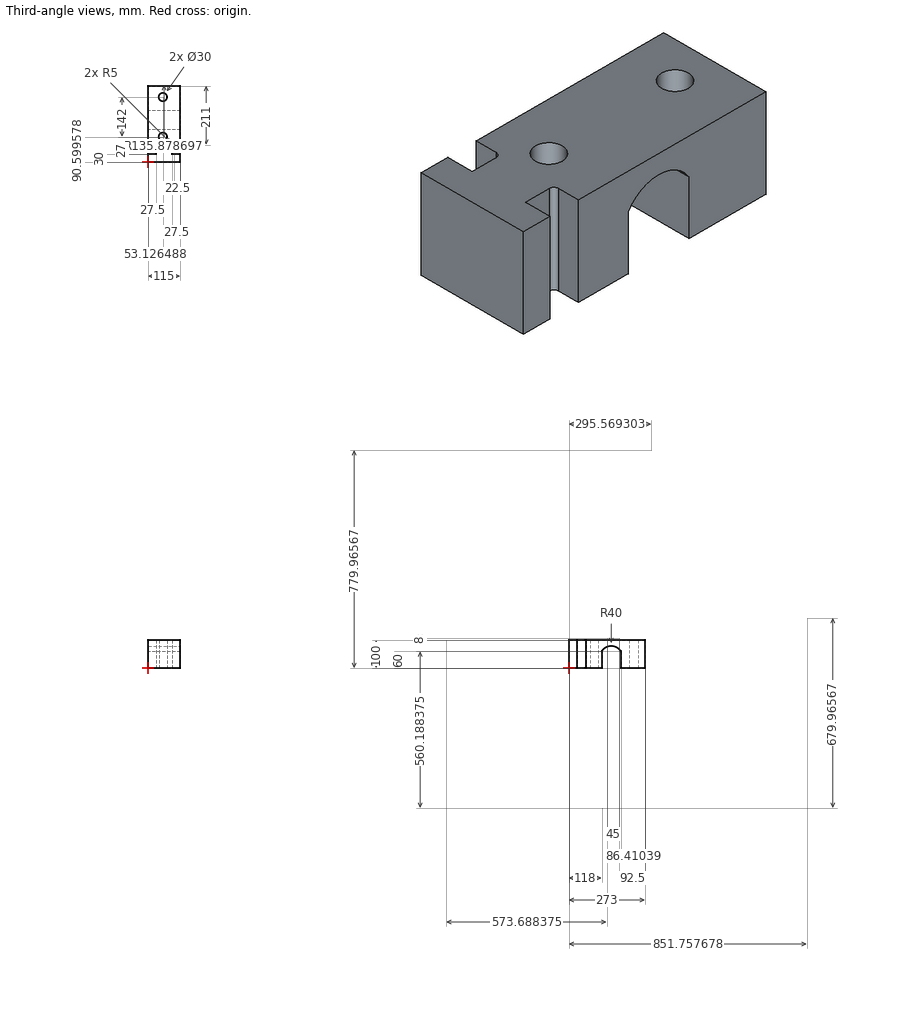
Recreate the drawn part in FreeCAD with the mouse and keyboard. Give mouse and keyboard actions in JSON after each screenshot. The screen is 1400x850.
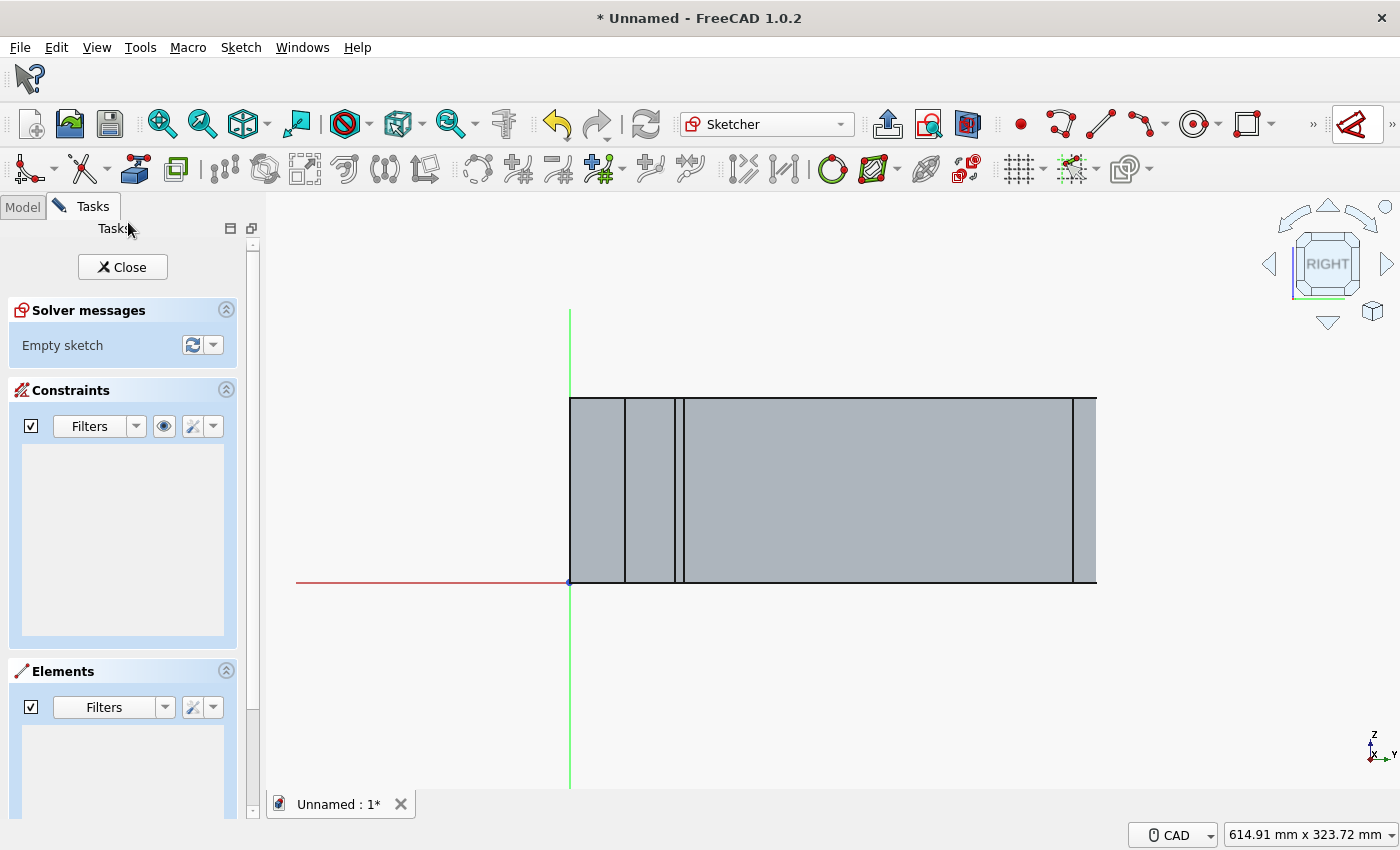
{"action": "key", "text": "q s"}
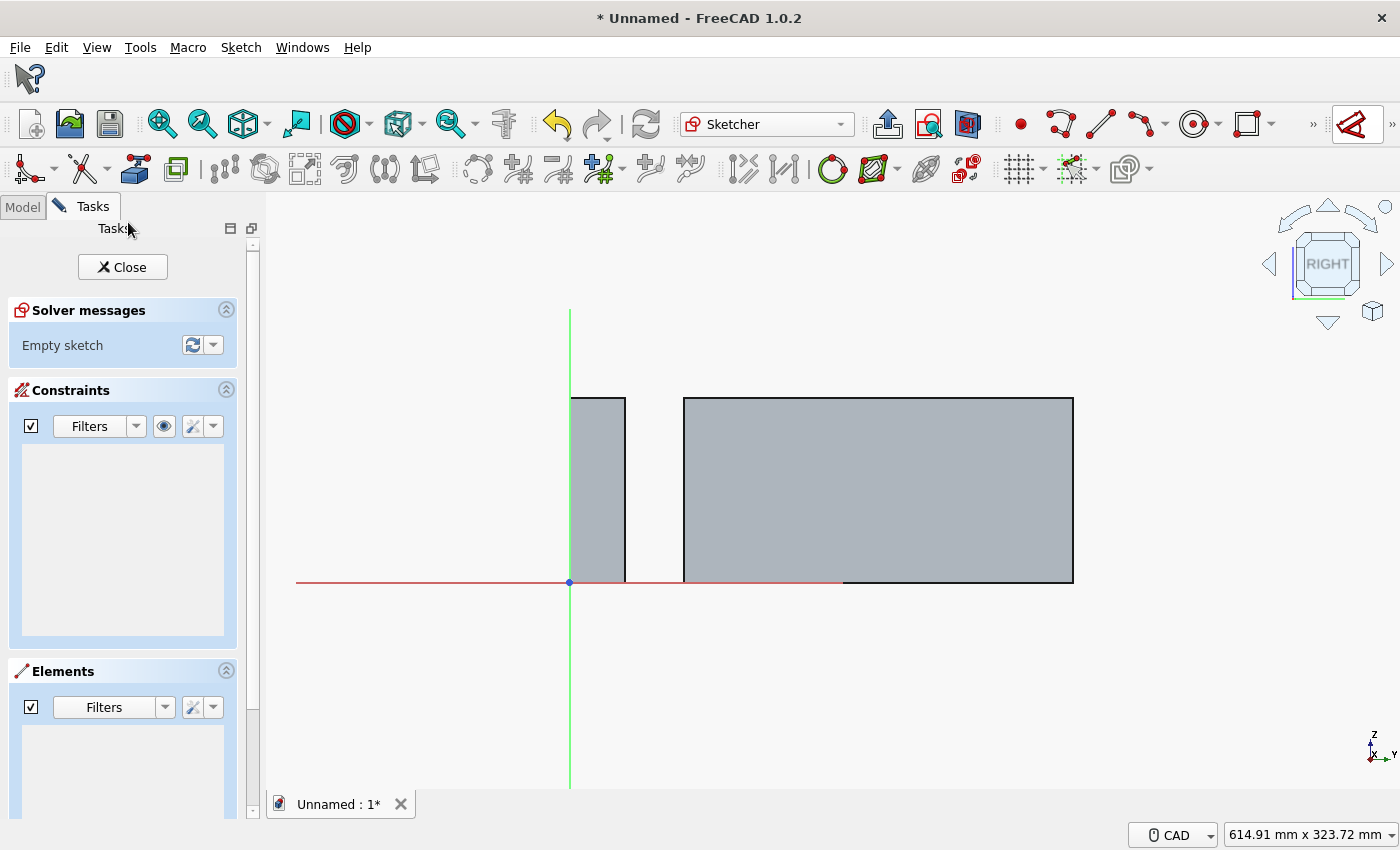
{"action": "scroll", "coordinate": [728, 523], "scroll_direction": "down", "scroll_amount": 9}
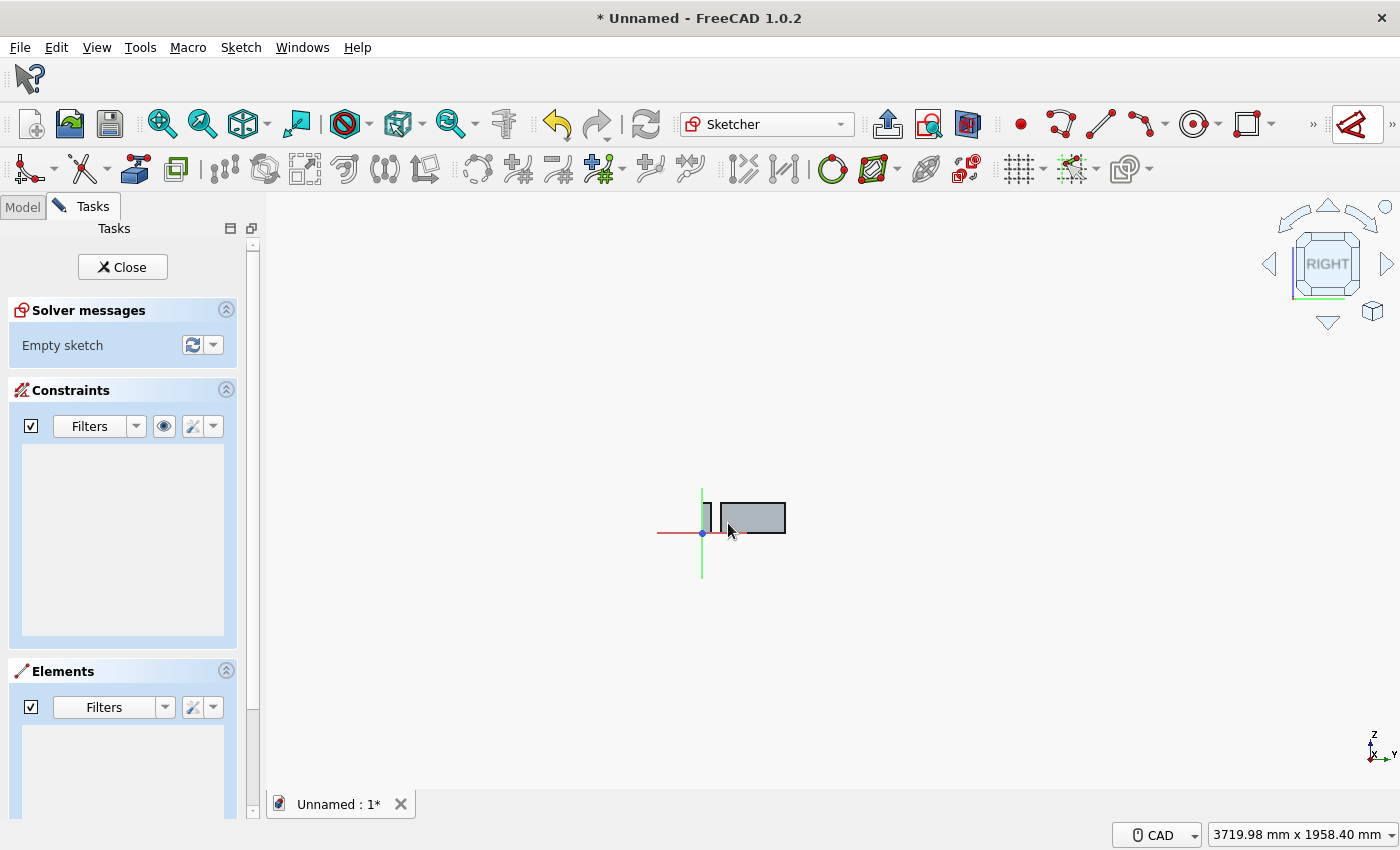
{"action": "key", "text": "g m"}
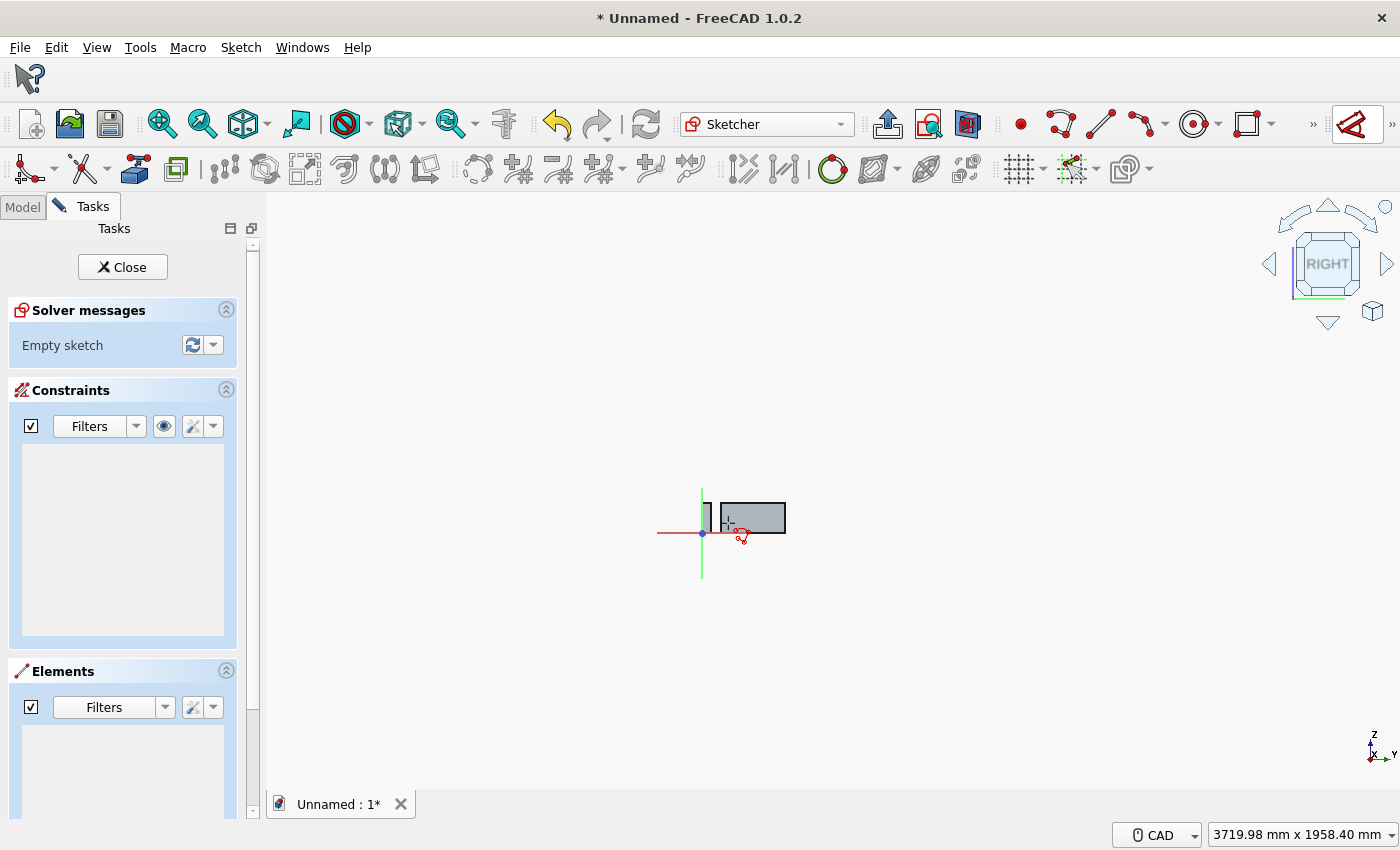
{"action": "left_click", "coordinate": [759, 515]}
{"action": "left_click", "coordinate": [759, 533]}
{"action": "left_click", "coordinate": [785, 524]}
{"action": "left_click", "coordinate": [785, 503]}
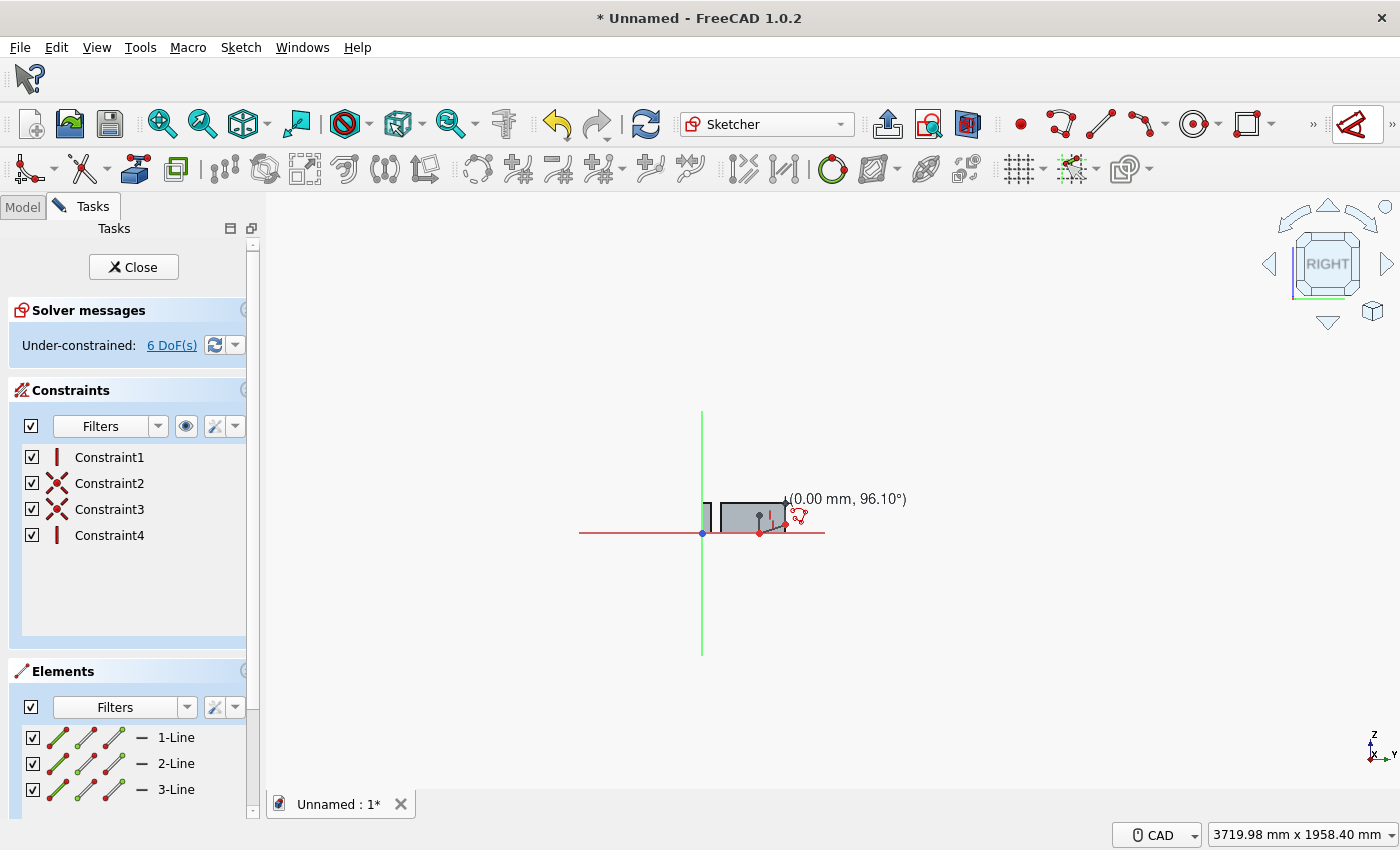
{"action": "scroll", "coordinate": [757, 503], "scroll_direction": "up", "scroll_amount": 2}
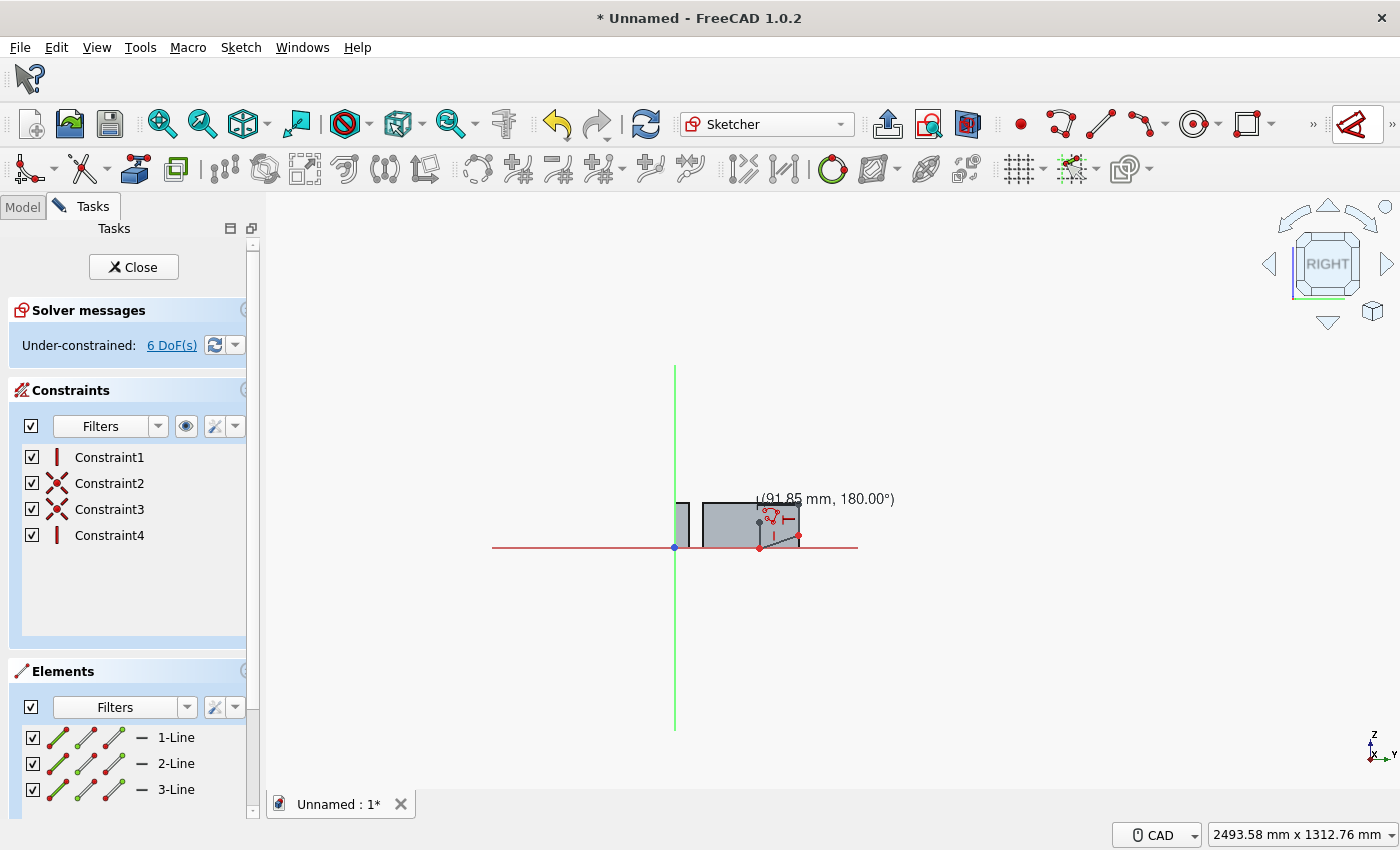
{"action": "left_click", "coordinate": [757, 503]}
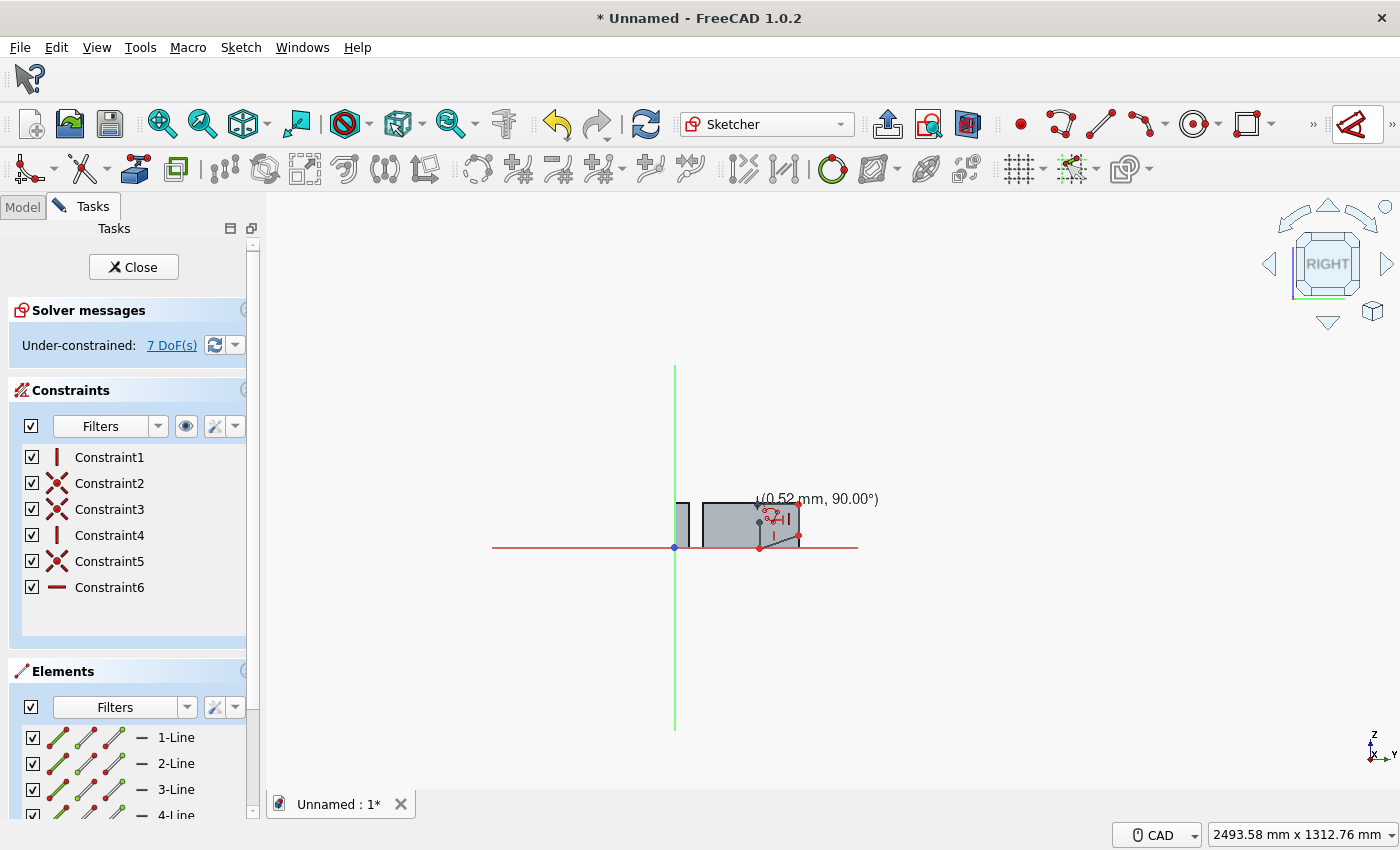
{"action": "scroll", "coordinate": [757, 499], "scroll_direction": "up", "scroll_amount": 8}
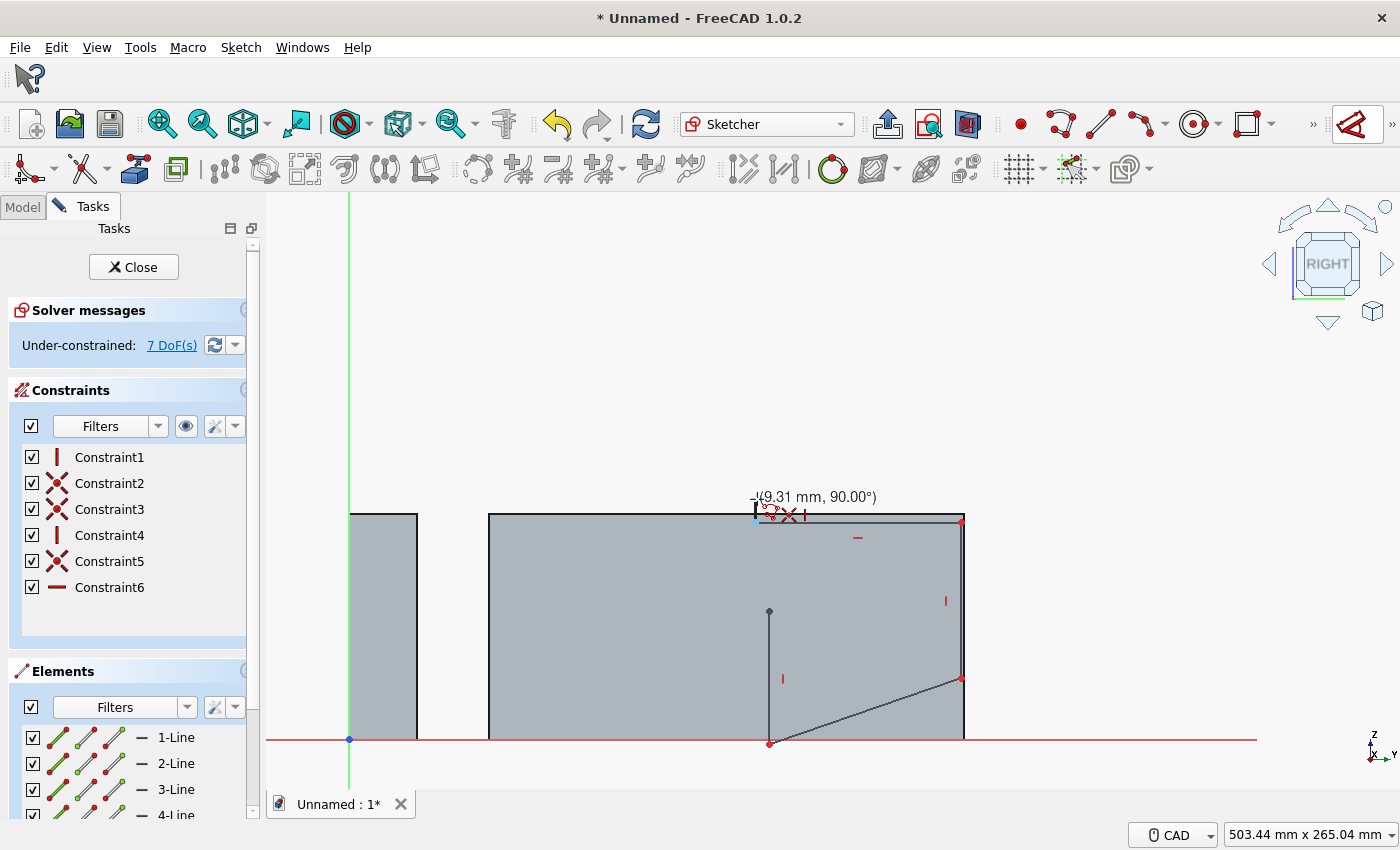
{"action": "left_click", "coordinate": [755, 496]}